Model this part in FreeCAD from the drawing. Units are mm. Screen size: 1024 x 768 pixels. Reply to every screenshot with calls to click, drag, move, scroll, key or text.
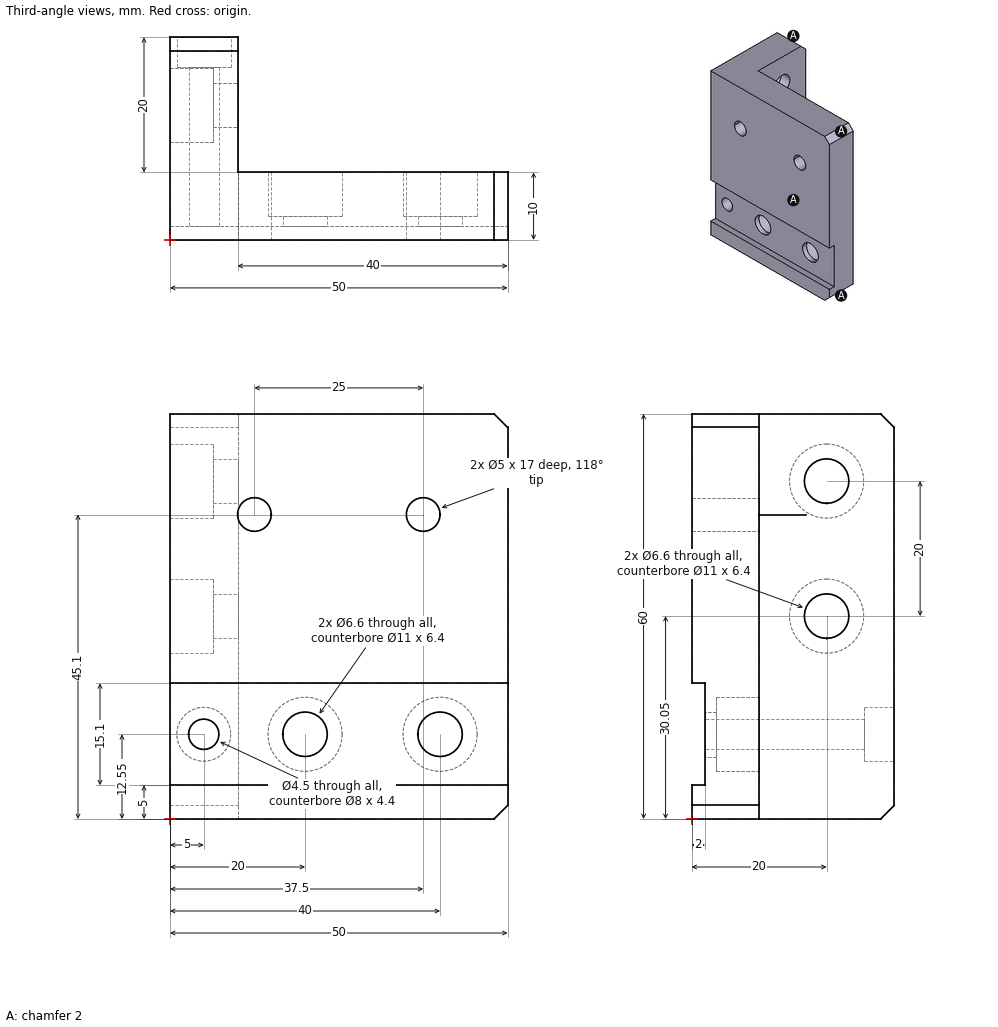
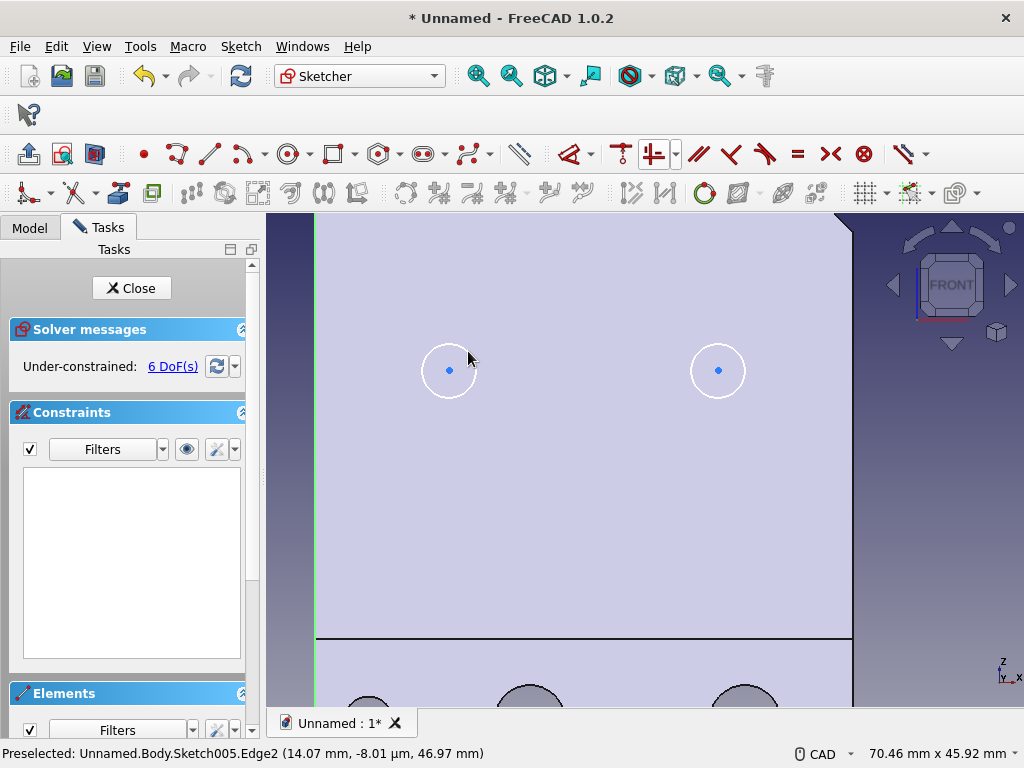
click(737, 352)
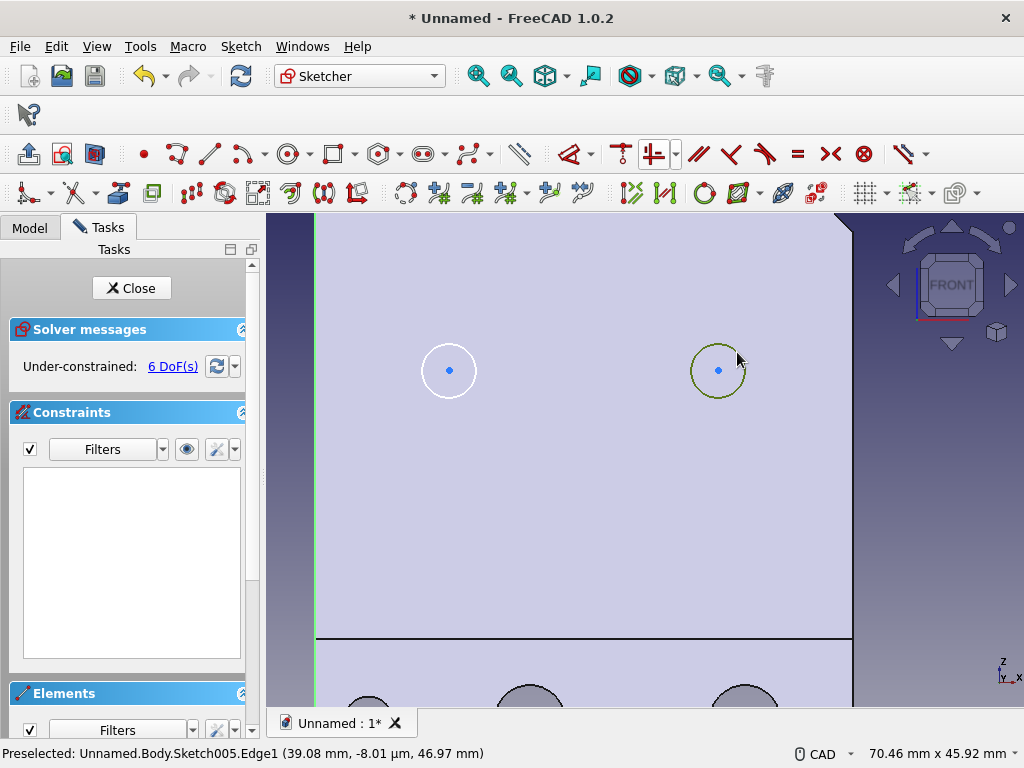
click(468, 352)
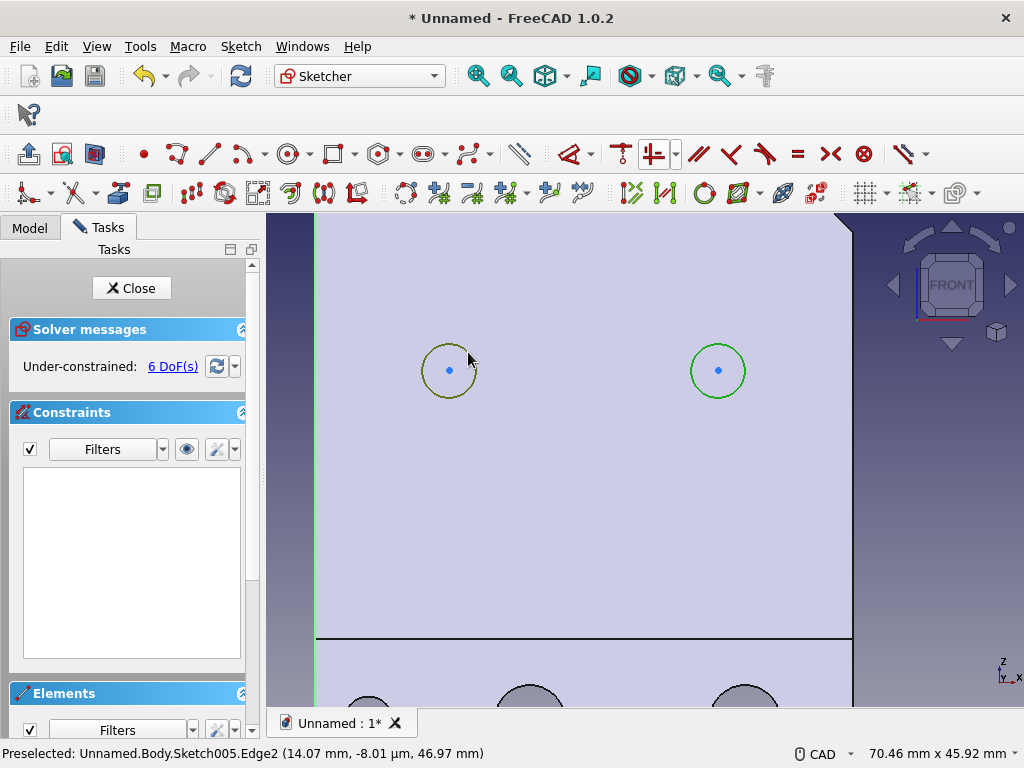
click(798, 154)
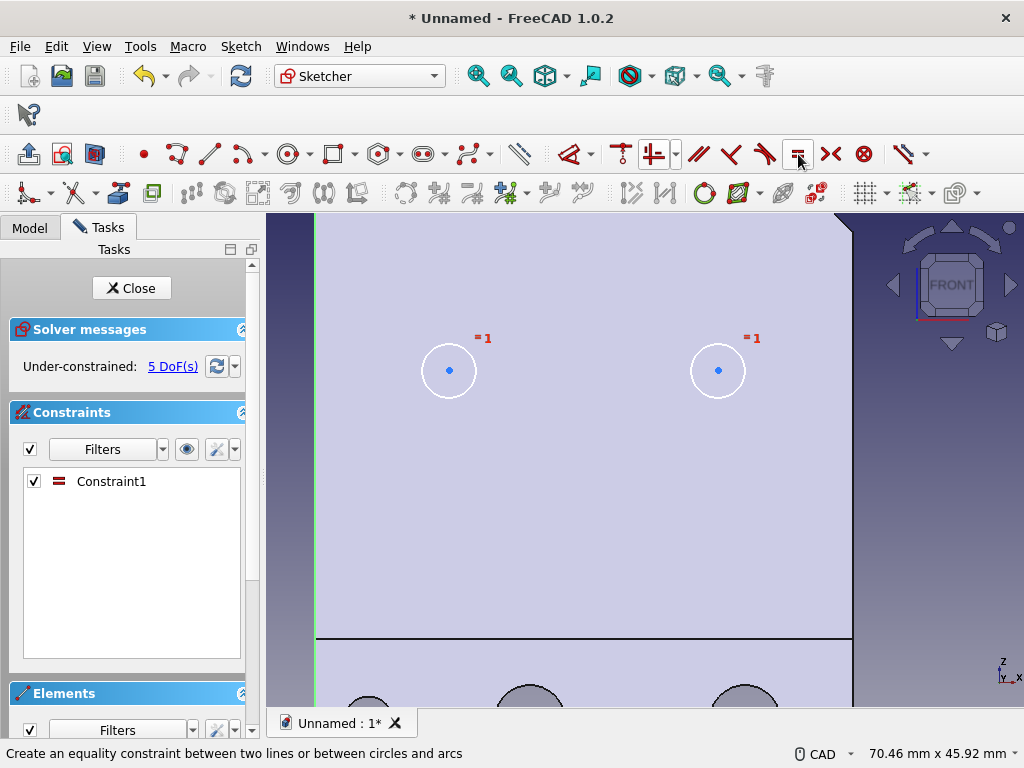
key(d)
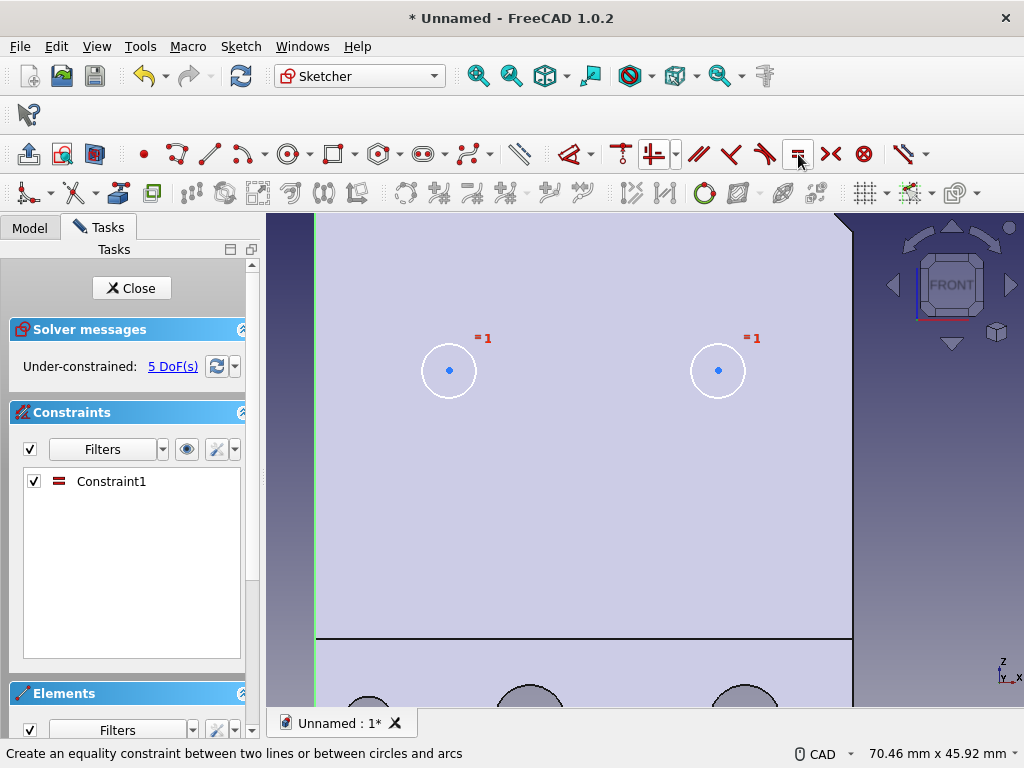
click(737, 352)
click(760, 329)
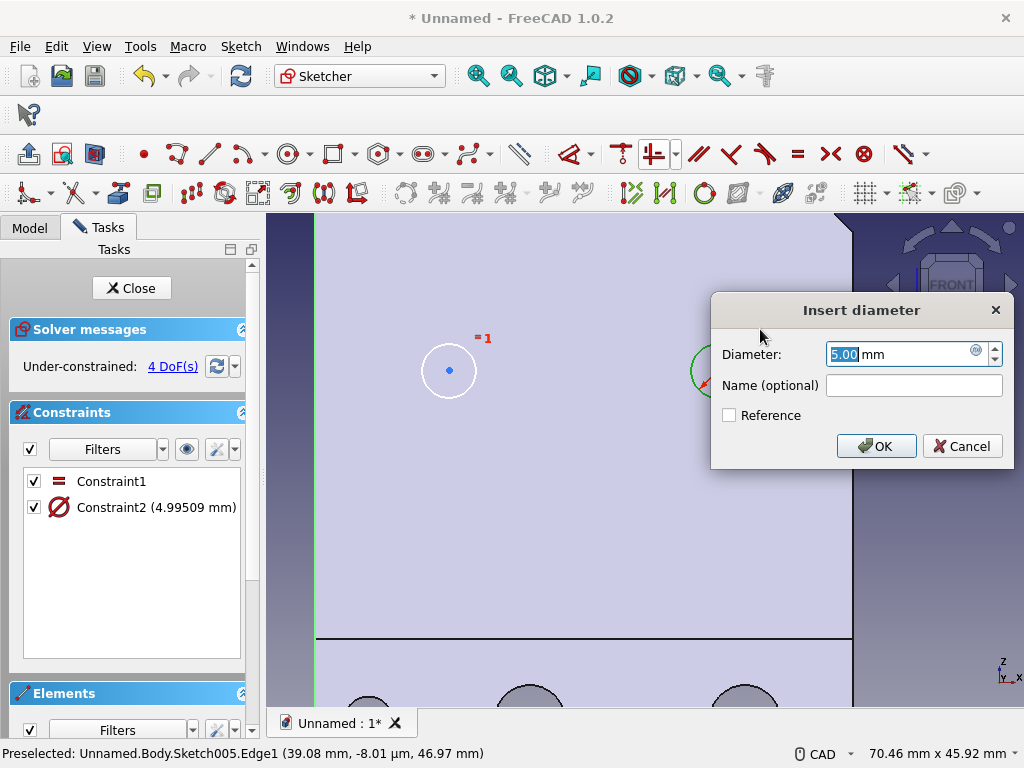
text(5)
key(Return)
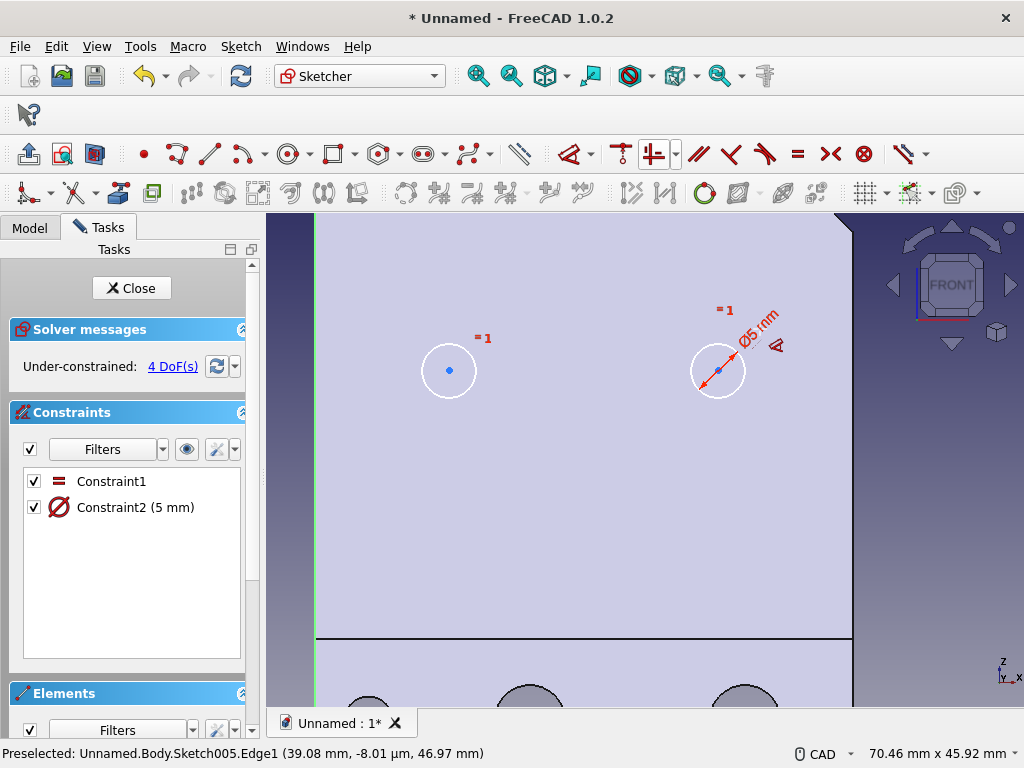
click(718, 371)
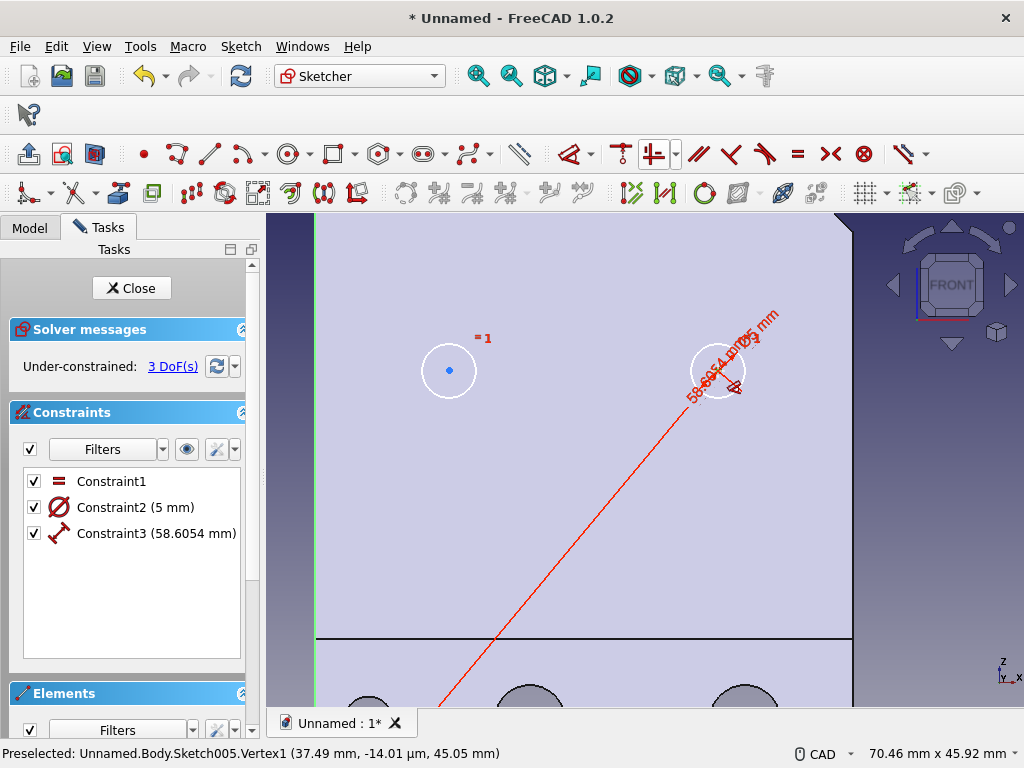
click(449, 371)
click(584, 337)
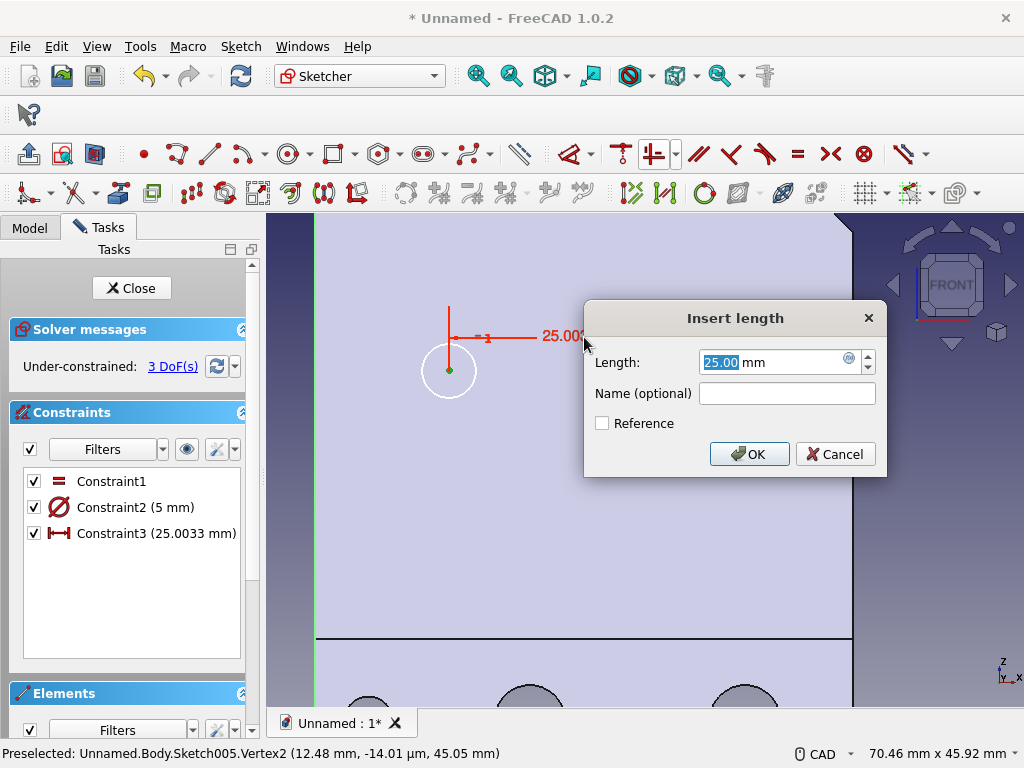
text(25)
key(Return)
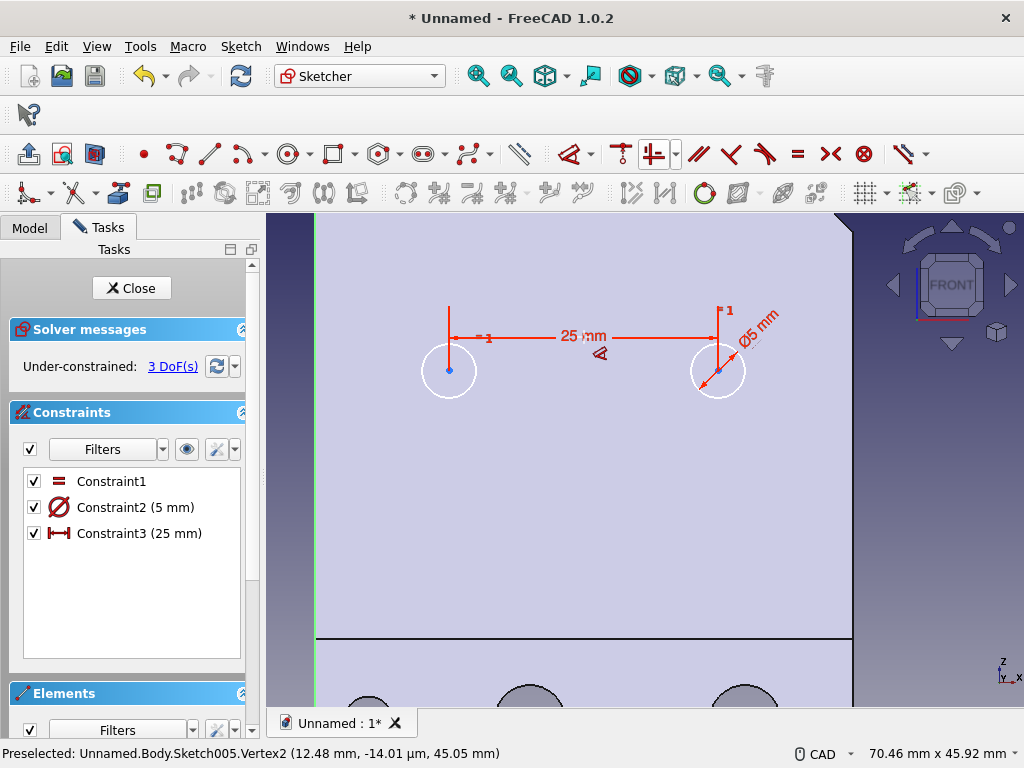
click(718, 371)
click(424, 337)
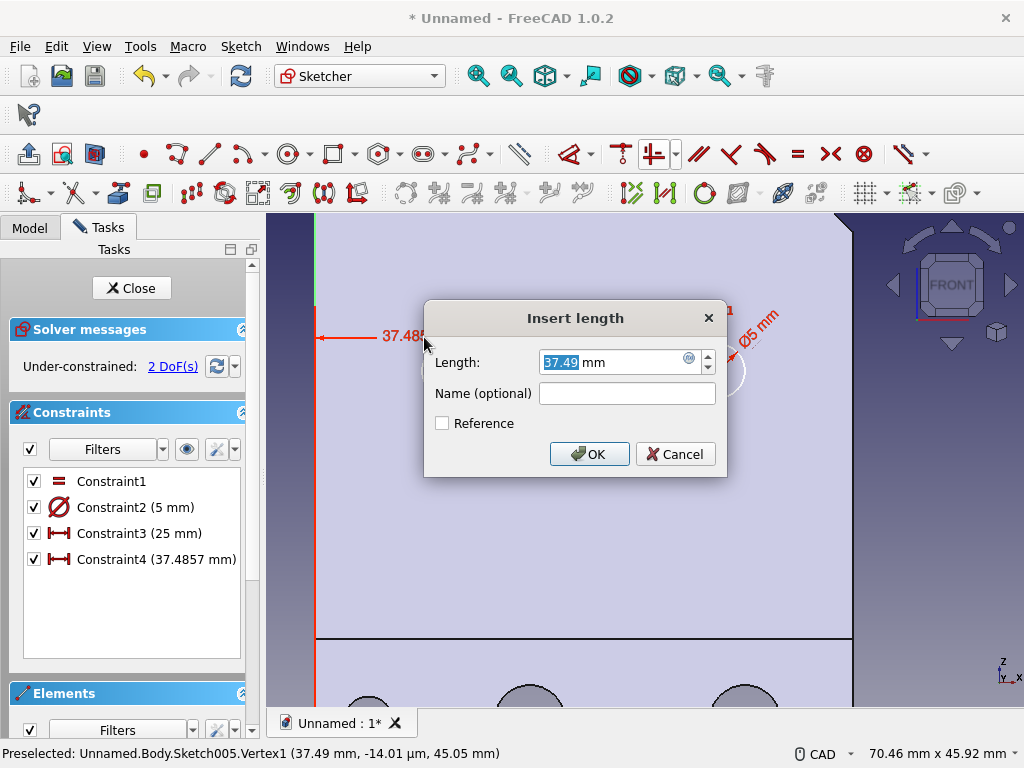
text(37.5)
key(Return)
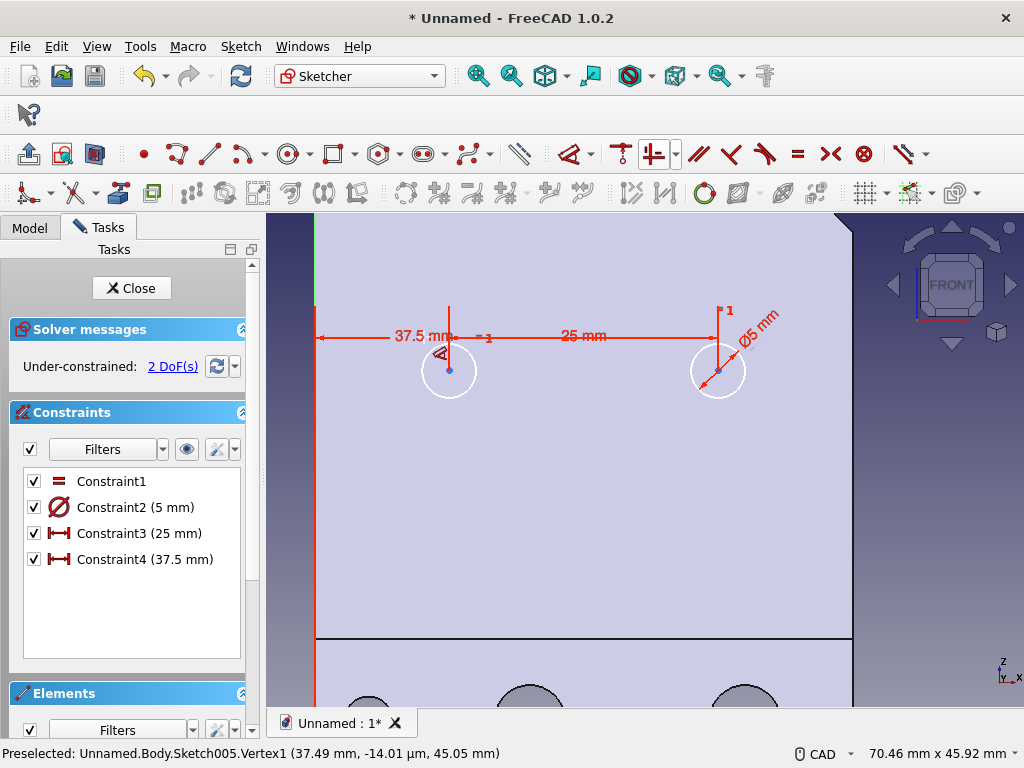
click(718, 371)
click(752, 525)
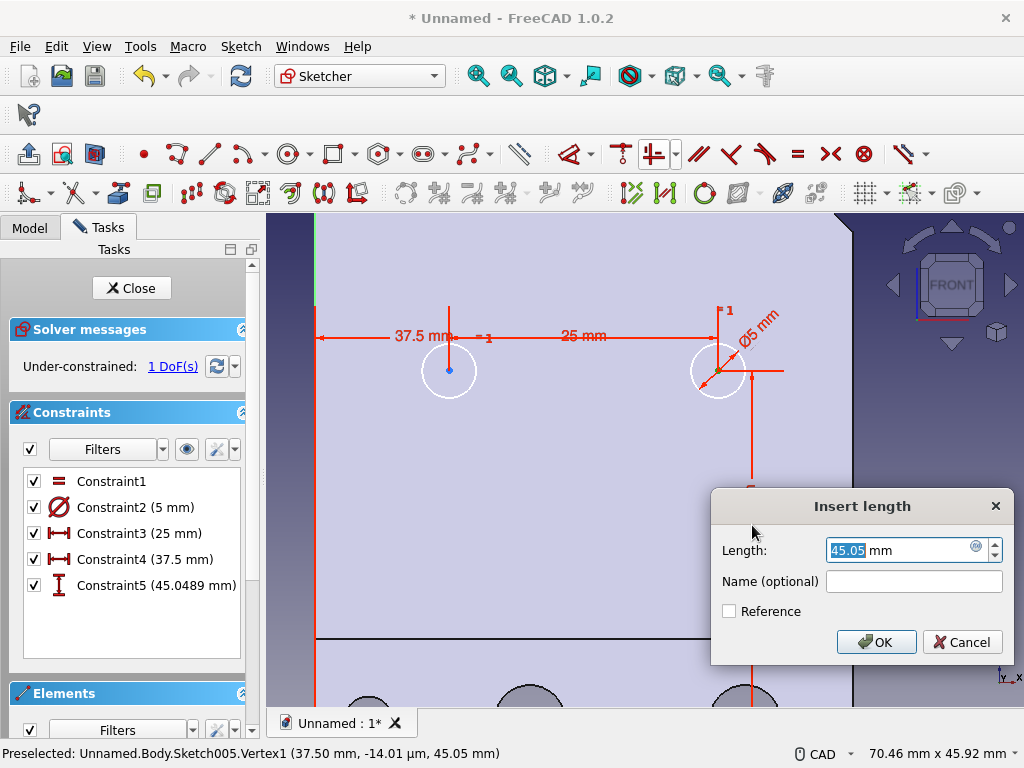
text(45.1)
key(Return)